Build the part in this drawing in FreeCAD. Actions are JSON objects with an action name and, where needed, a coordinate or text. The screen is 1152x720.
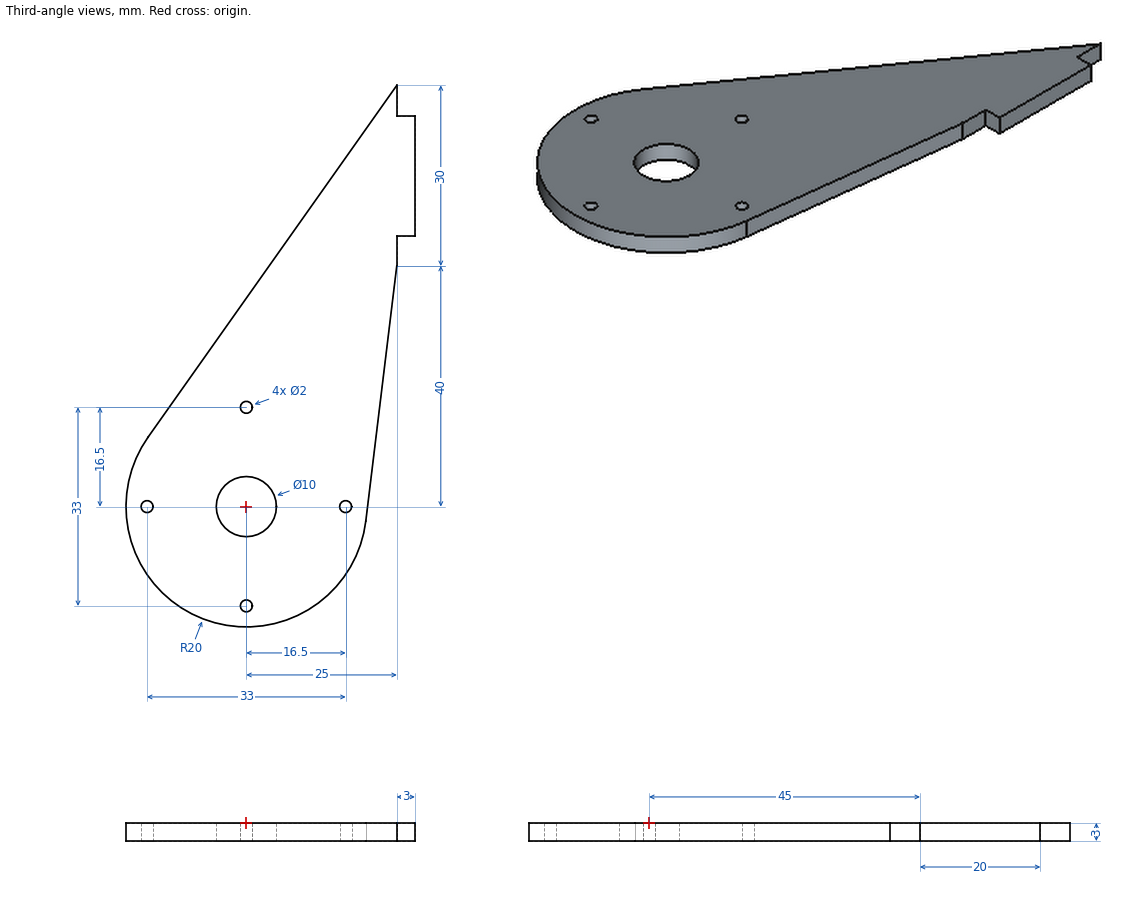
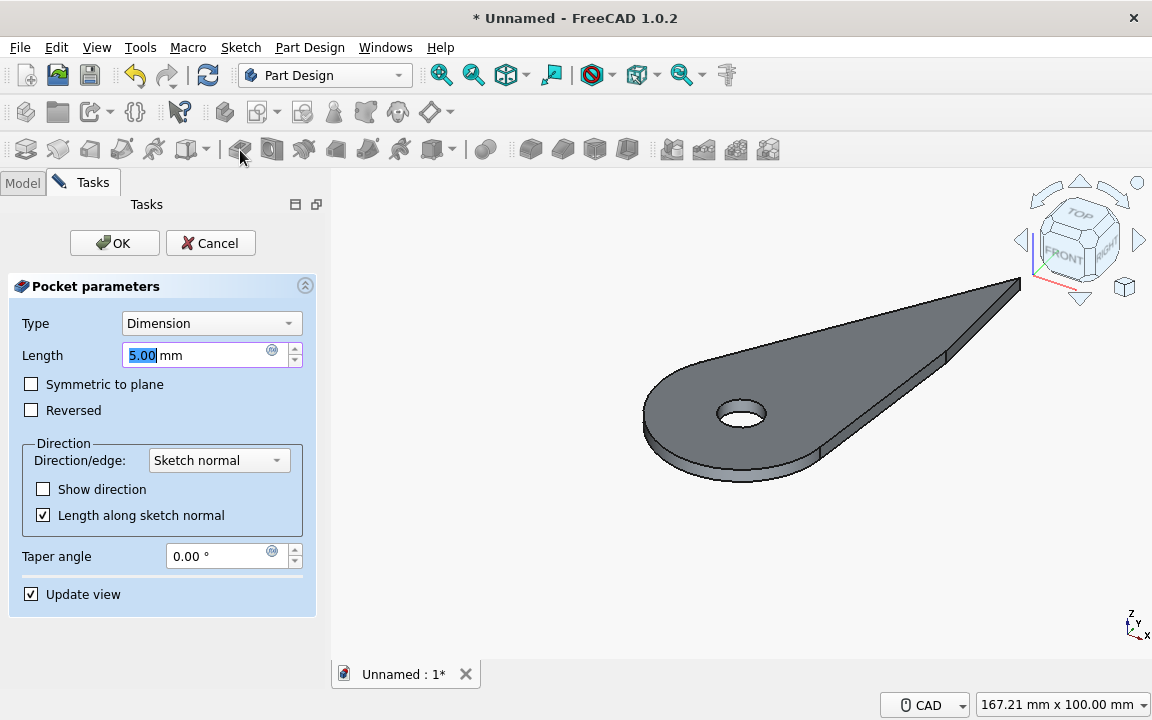
{"action": "type", "text": "10"}
{"action": "key", "text": "Tab"}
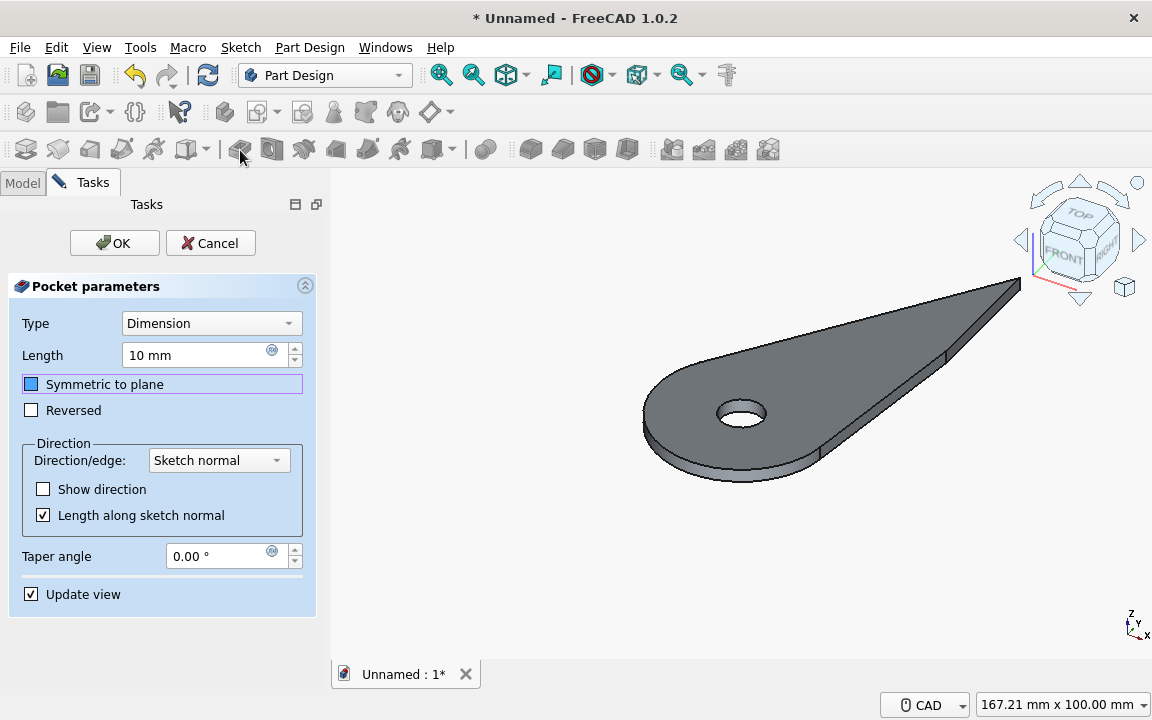
{"action": "left_click", "coordinate": [115, 243]}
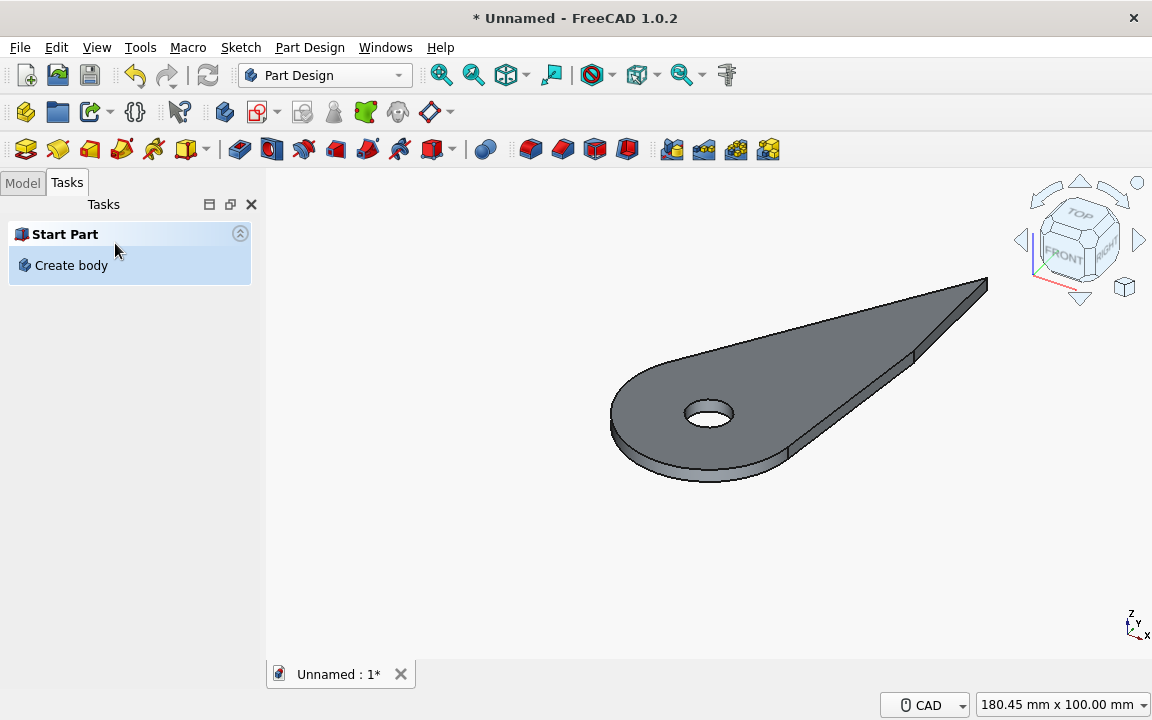
{"action": "key", "text": "0"}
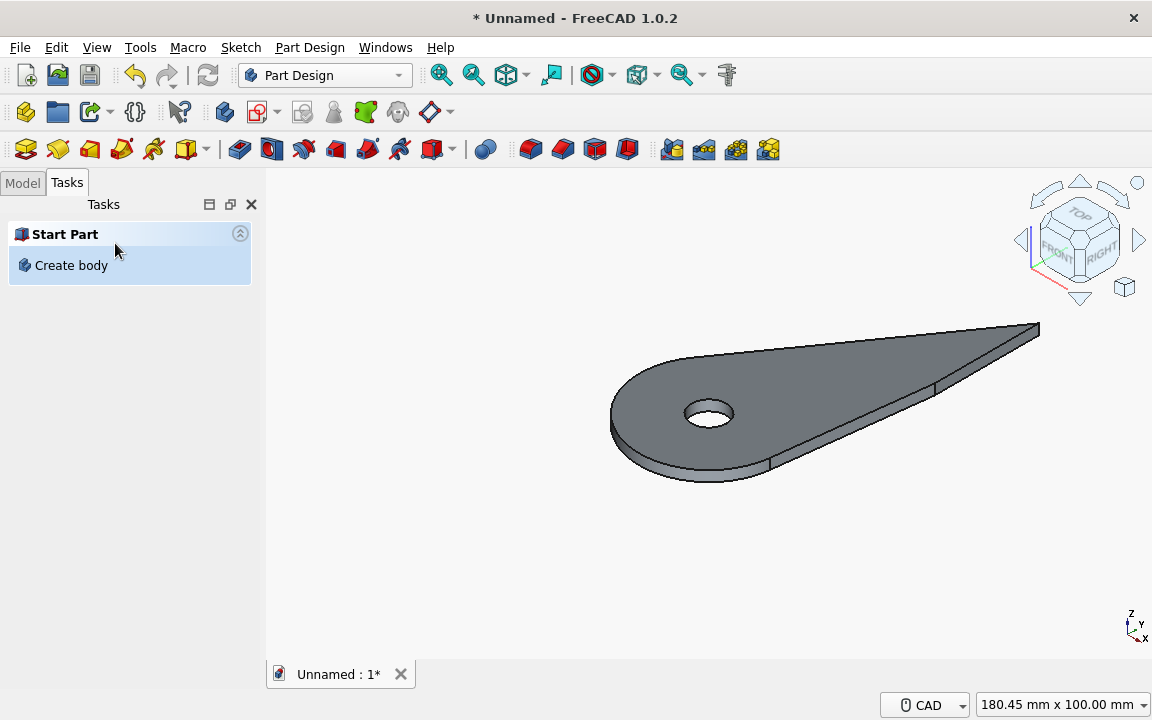
{"action": "key", "text": "3"}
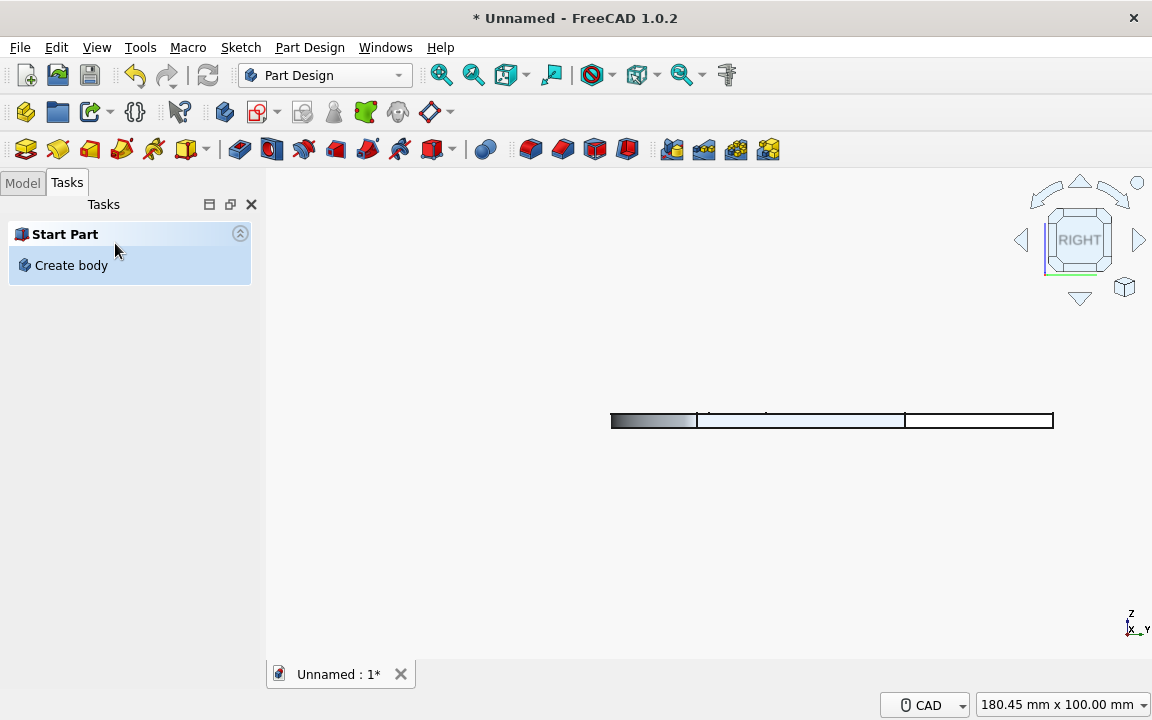
{"action": "key", "text": "2"}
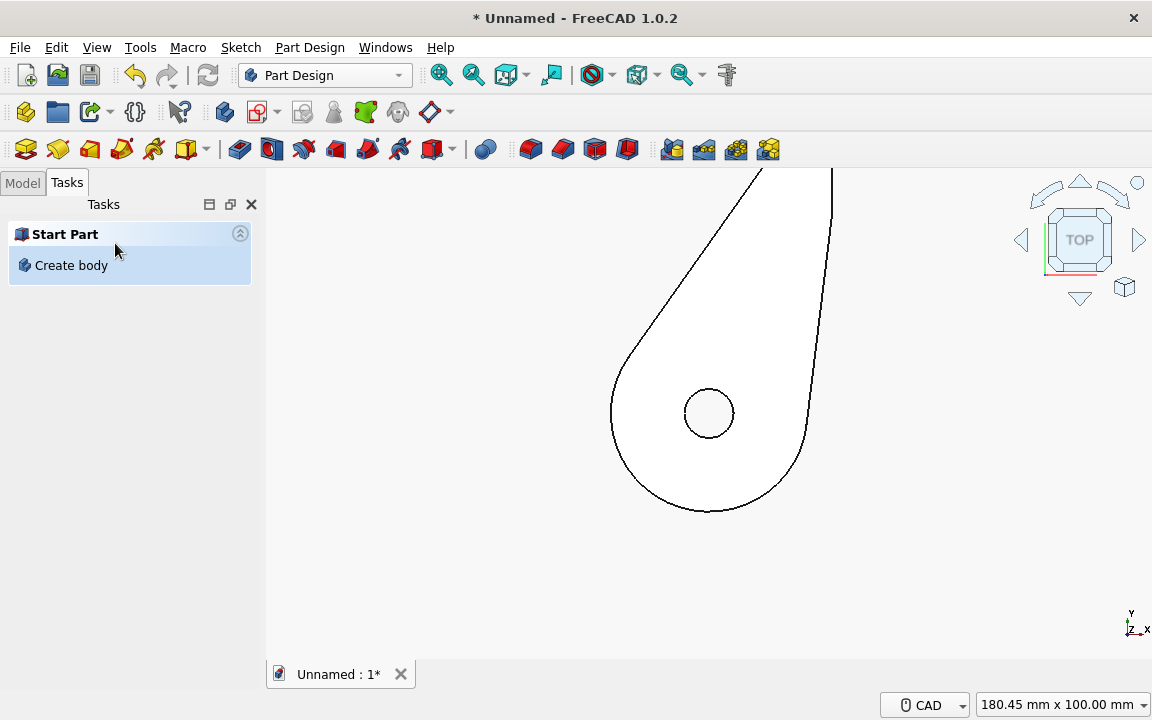
{"action": "left_click", "coordinate": [442, 76]}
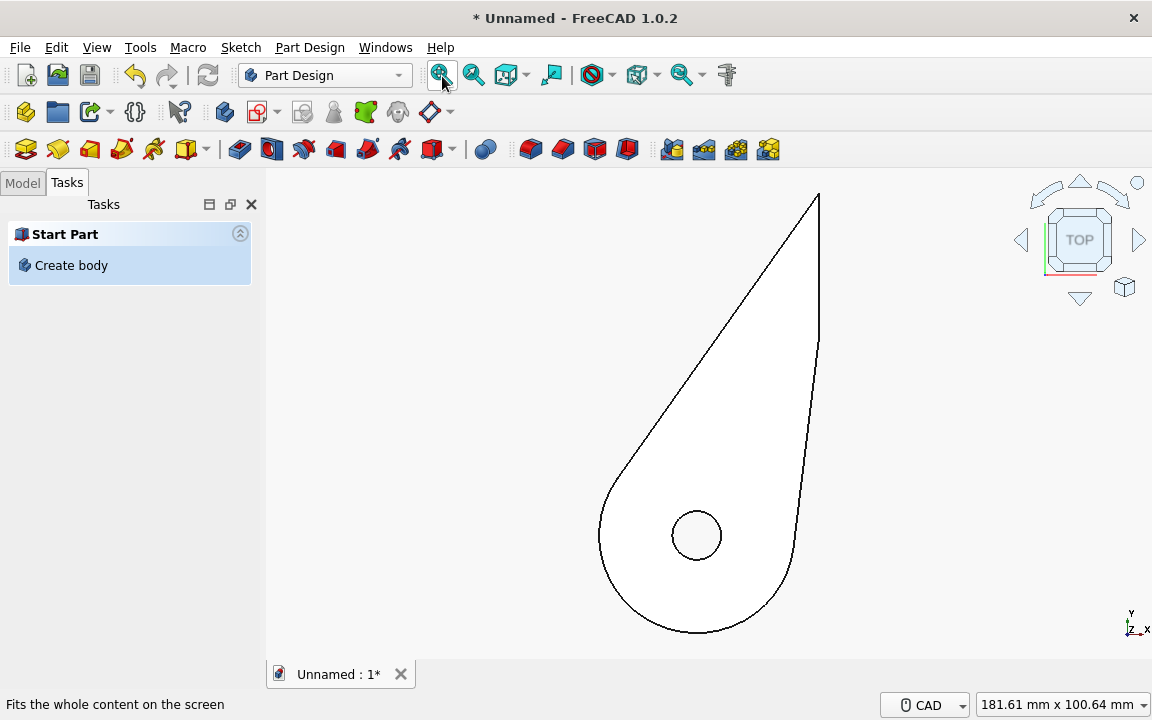
{"action": "left_click", "coordinate": [23, 182]}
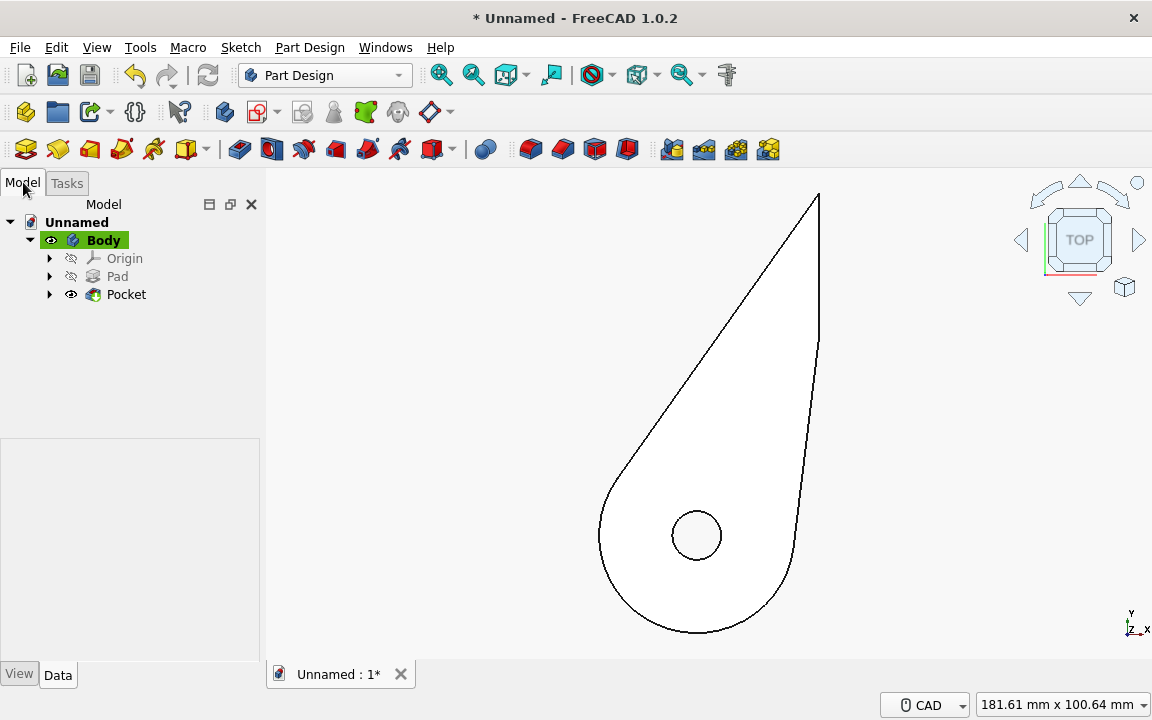
{"action": "left_click", "coordinate": [50, 258]}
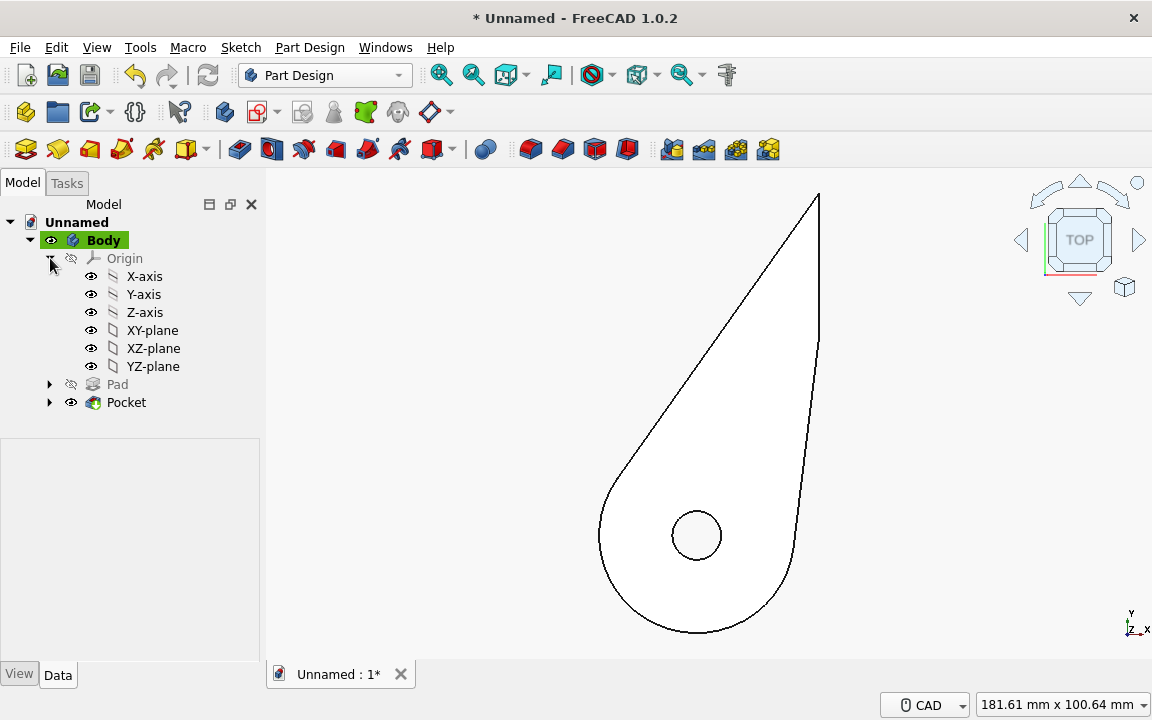
{"action": "left_click", "coordinate": [136, 366]}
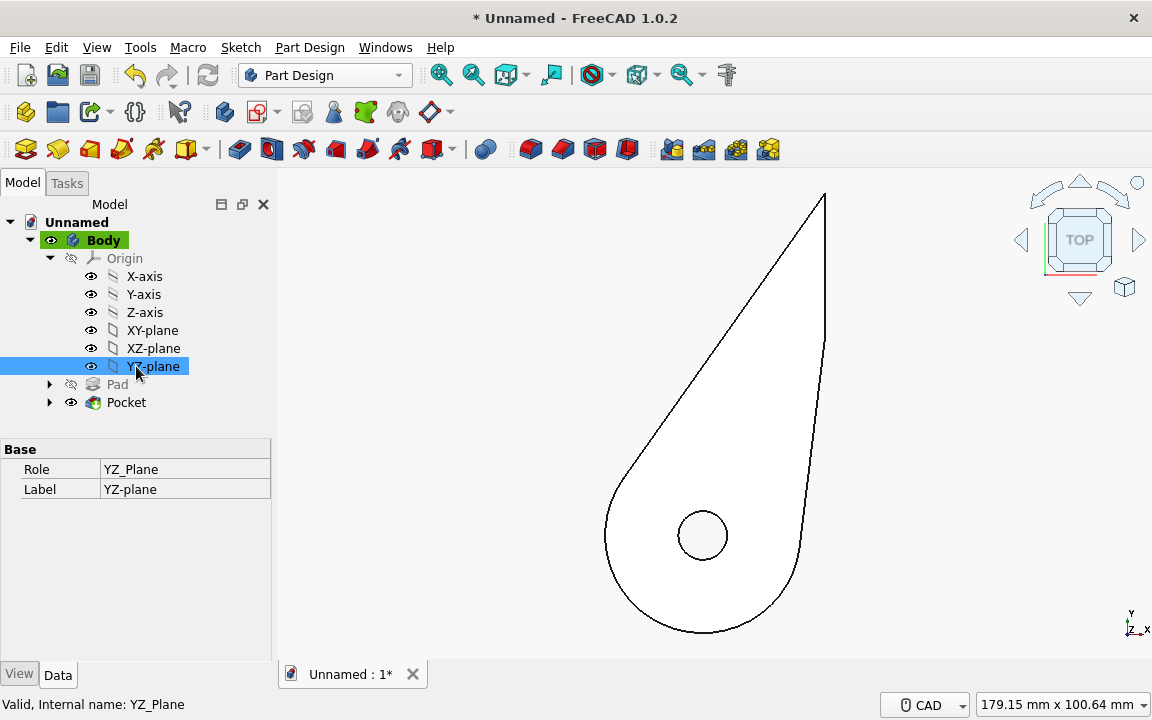
{"action": "left_click", "coordinate": [430, 112]}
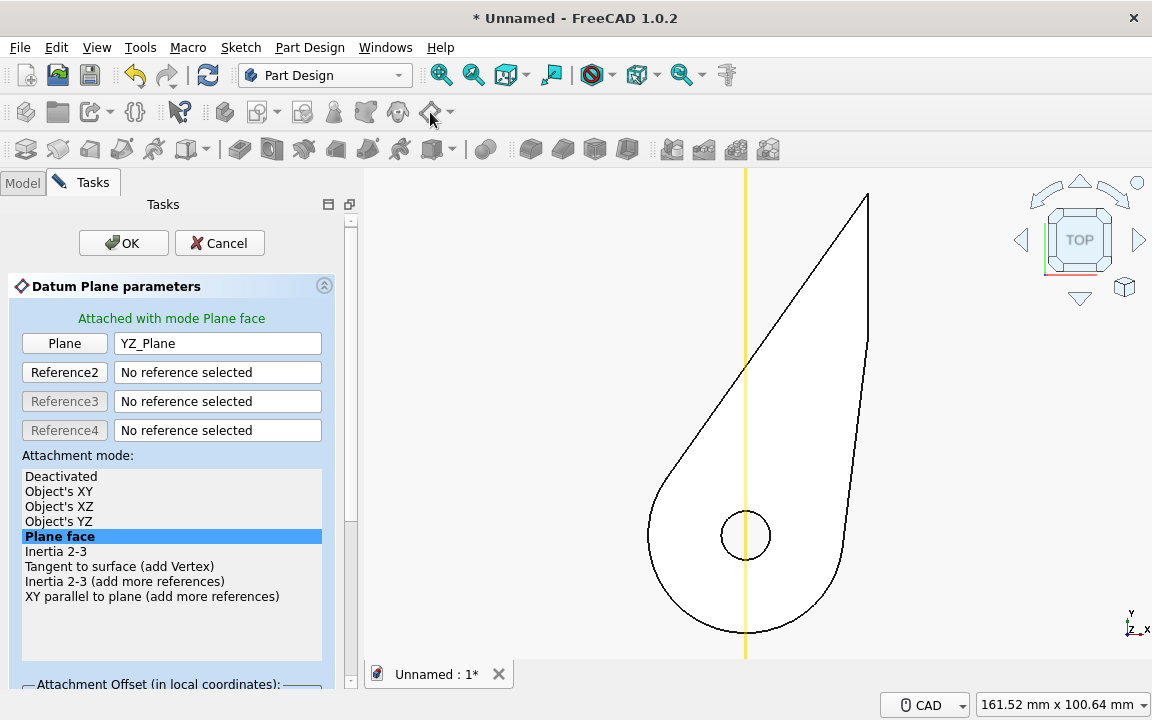
{"action": "scroll", "coordinate": [351, 451], "scroll_direction": "down", "scroll_amount": 3}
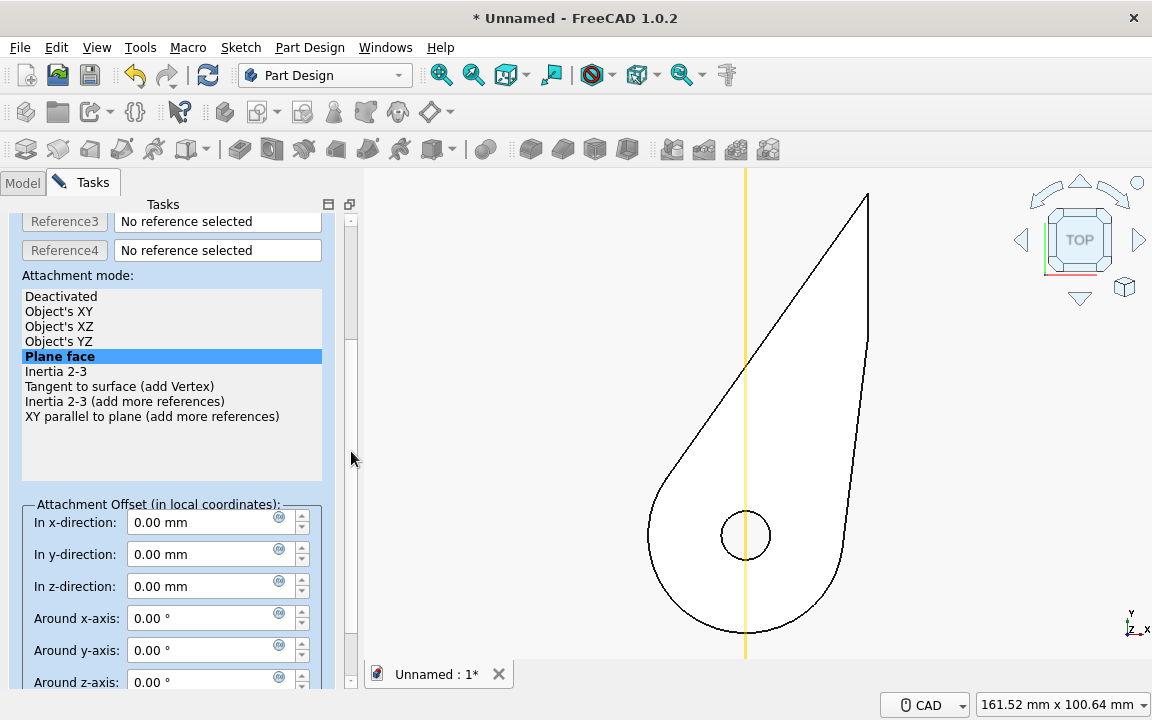
{"action": "triple_click", "coordinate": [210, 586]}